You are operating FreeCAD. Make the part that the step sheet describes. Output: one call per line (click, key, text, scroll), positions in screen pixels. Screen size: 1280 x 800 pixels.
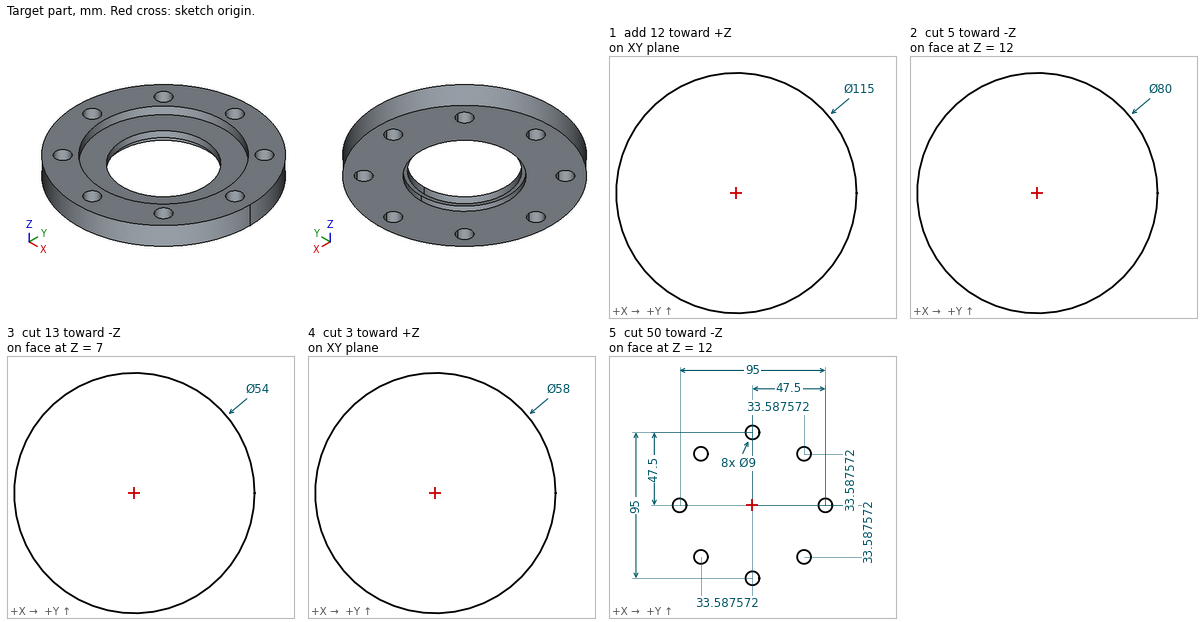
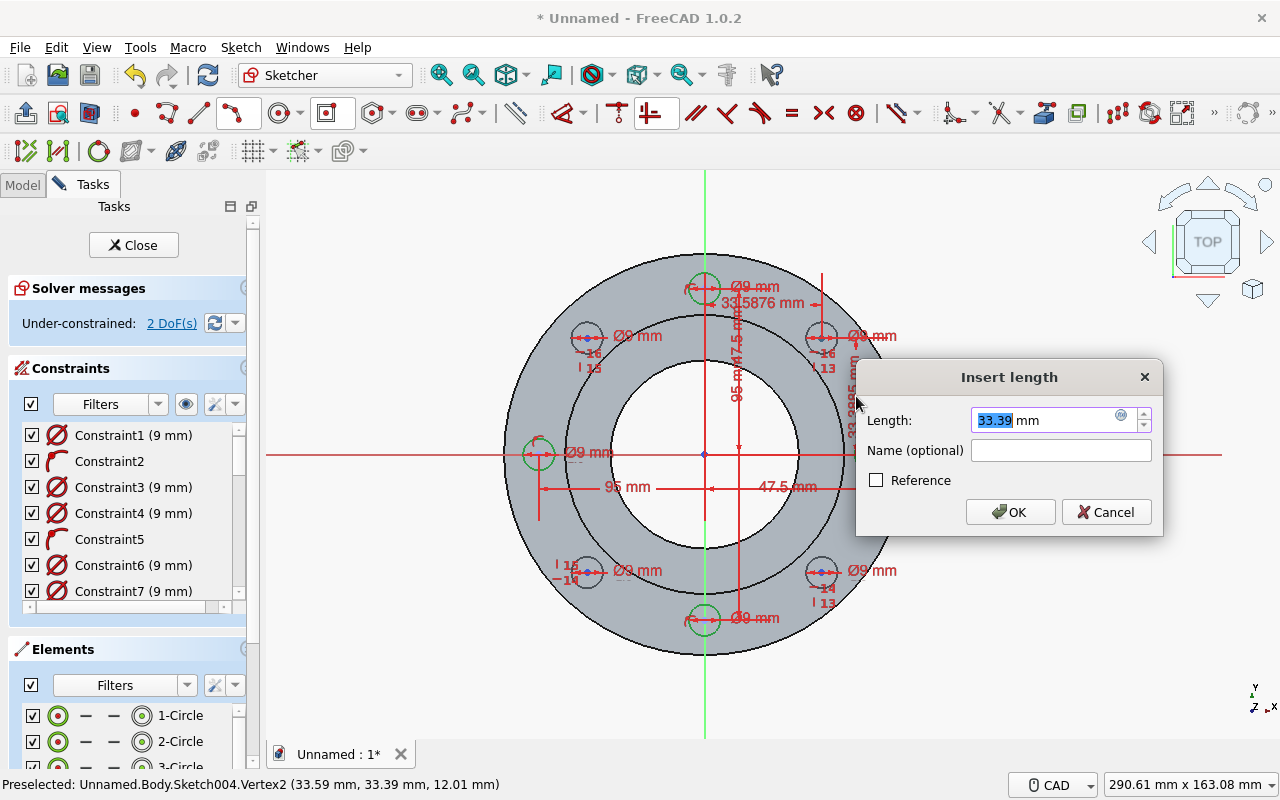
text(33.587572)
key(Return)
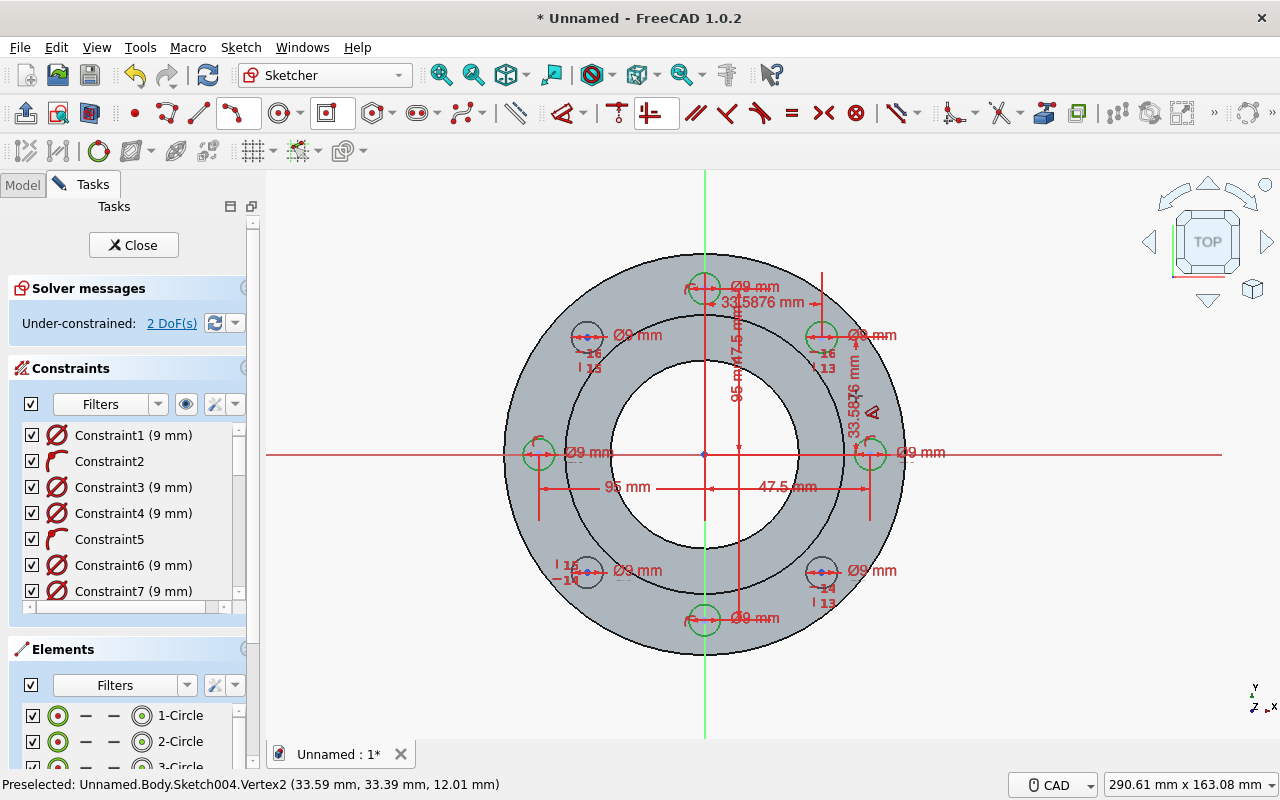
click(822, 573)
click(856, 514)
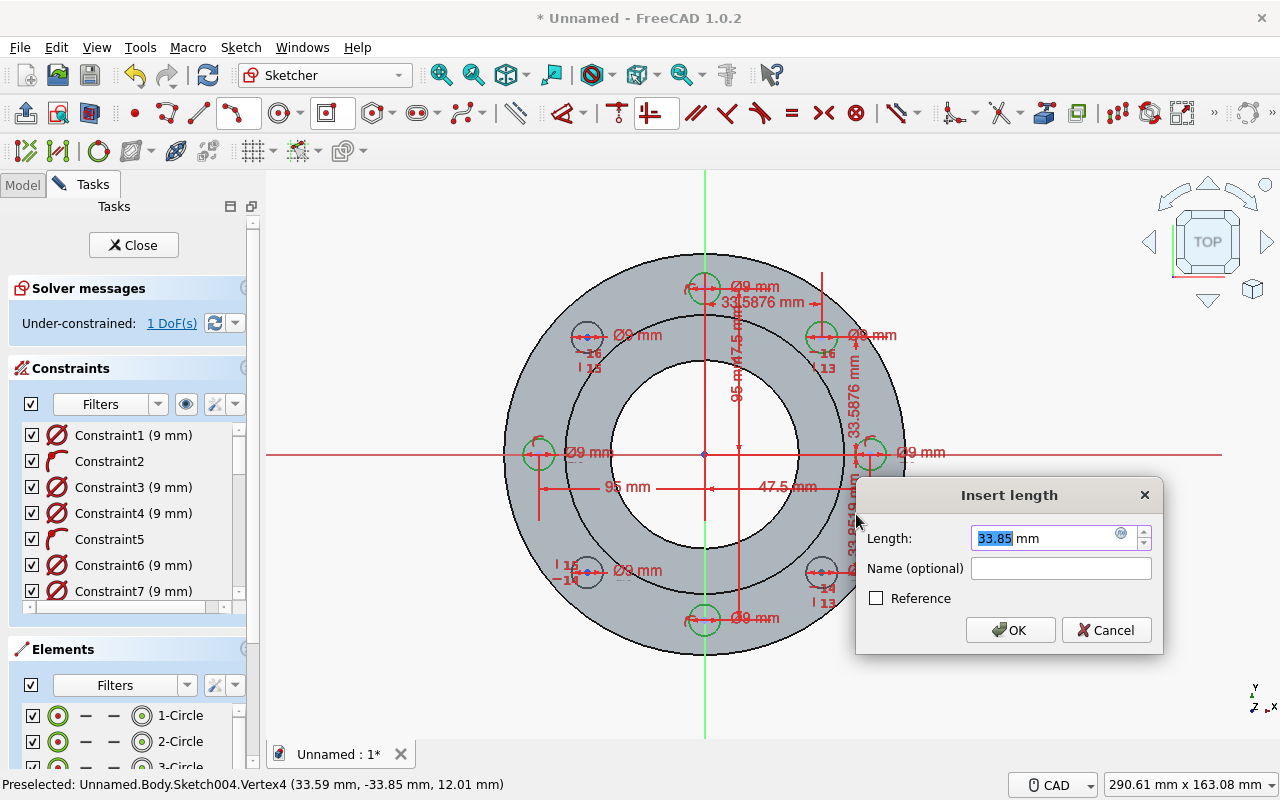
text(33.587572)
key(Return)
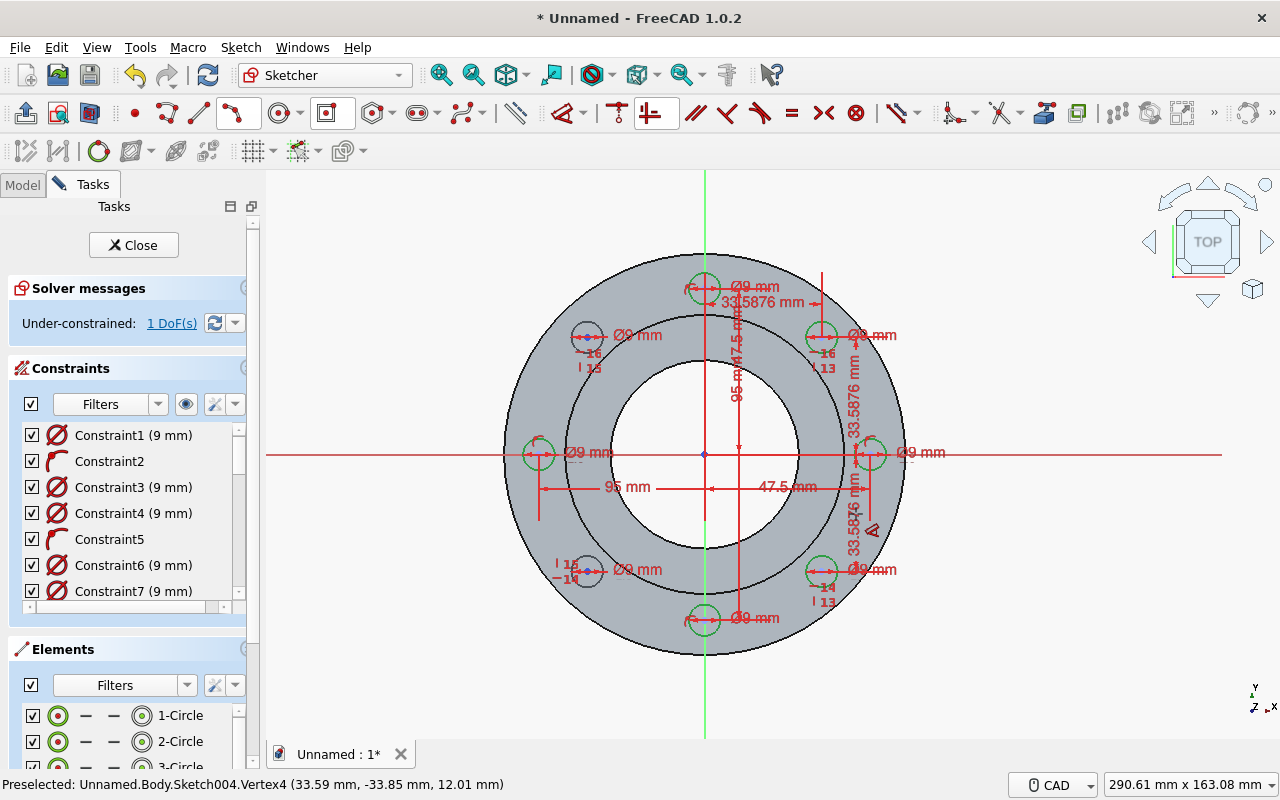
click(587, 572)
click(646, 606)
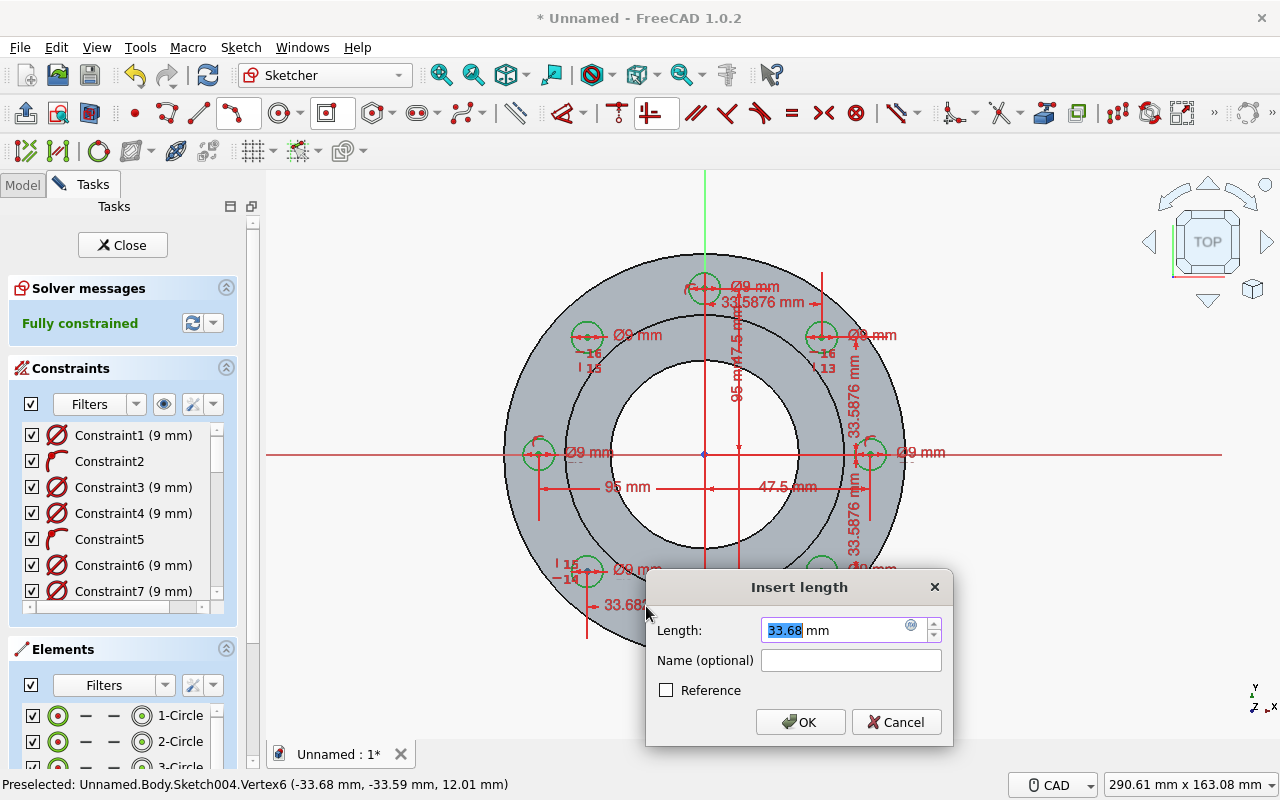
text(33.587572)
key(Return)
key(Escape)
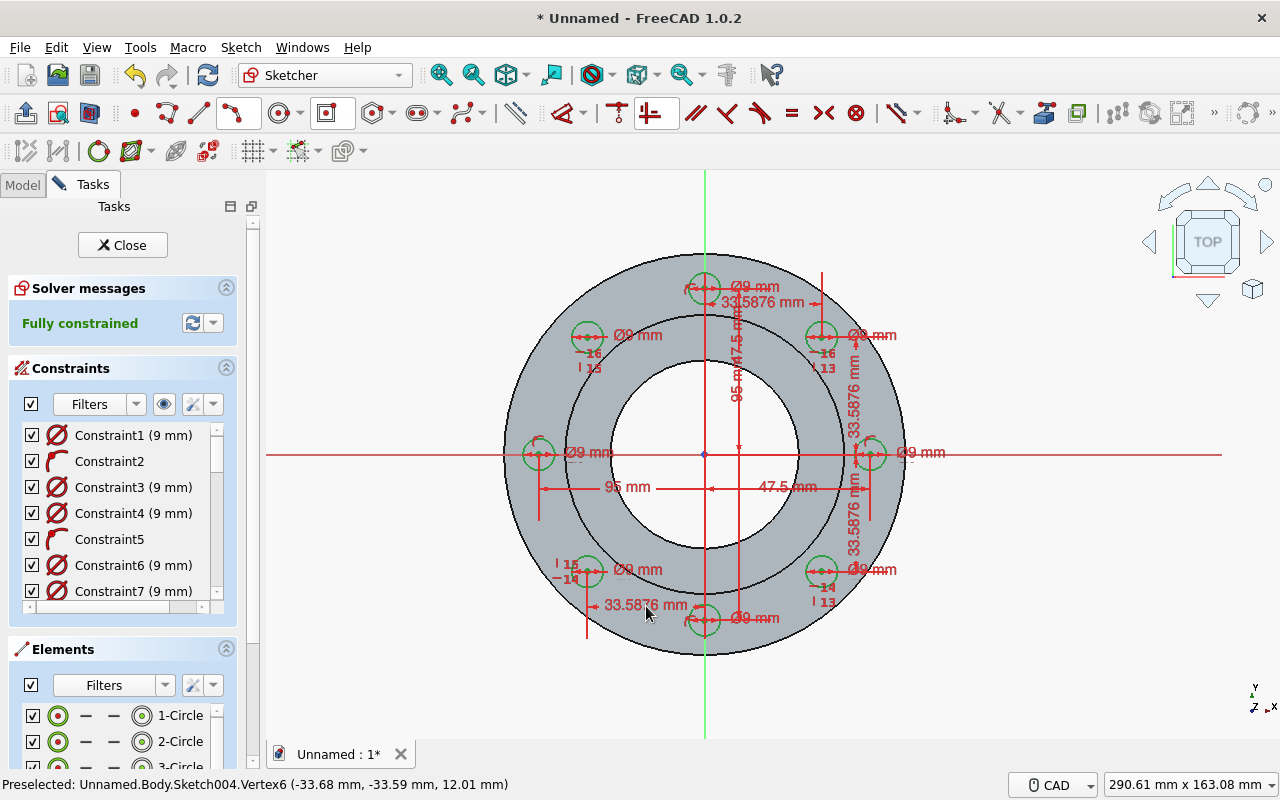
click(123, 245)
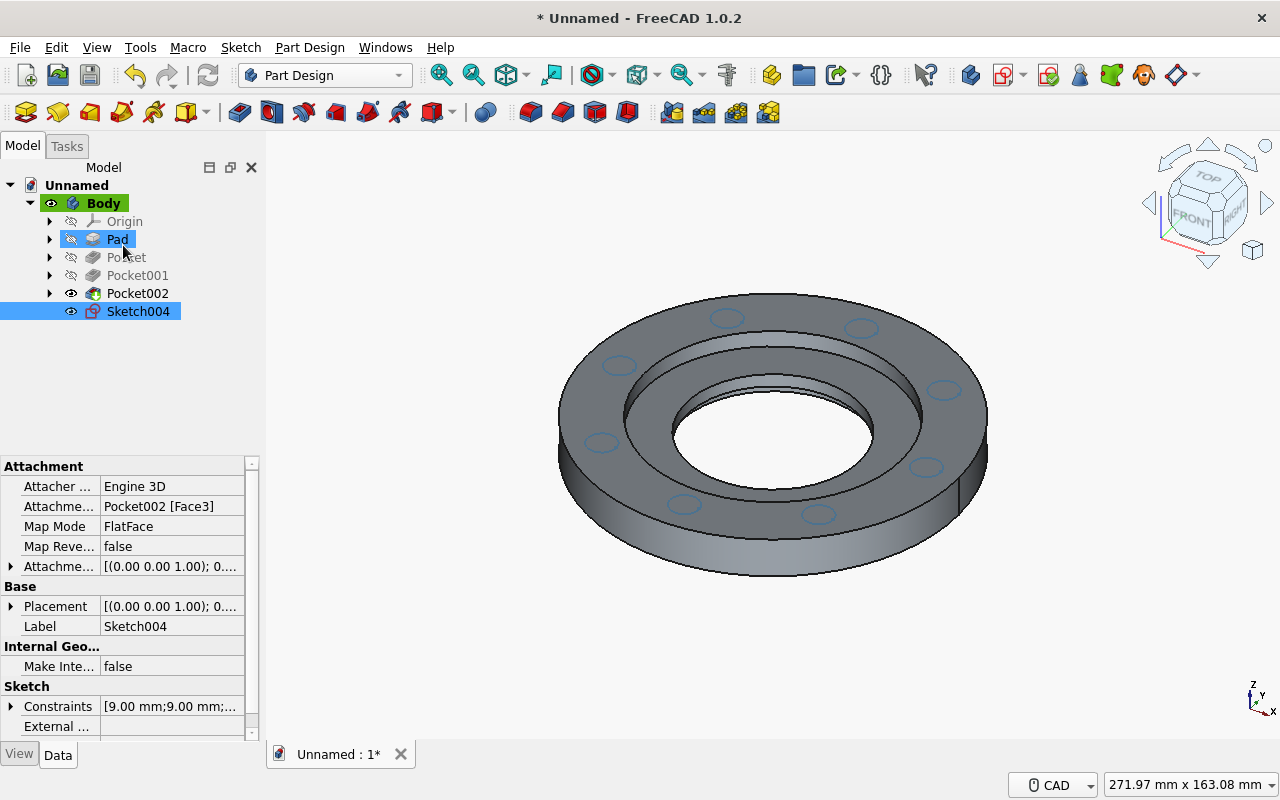
click(240, 112)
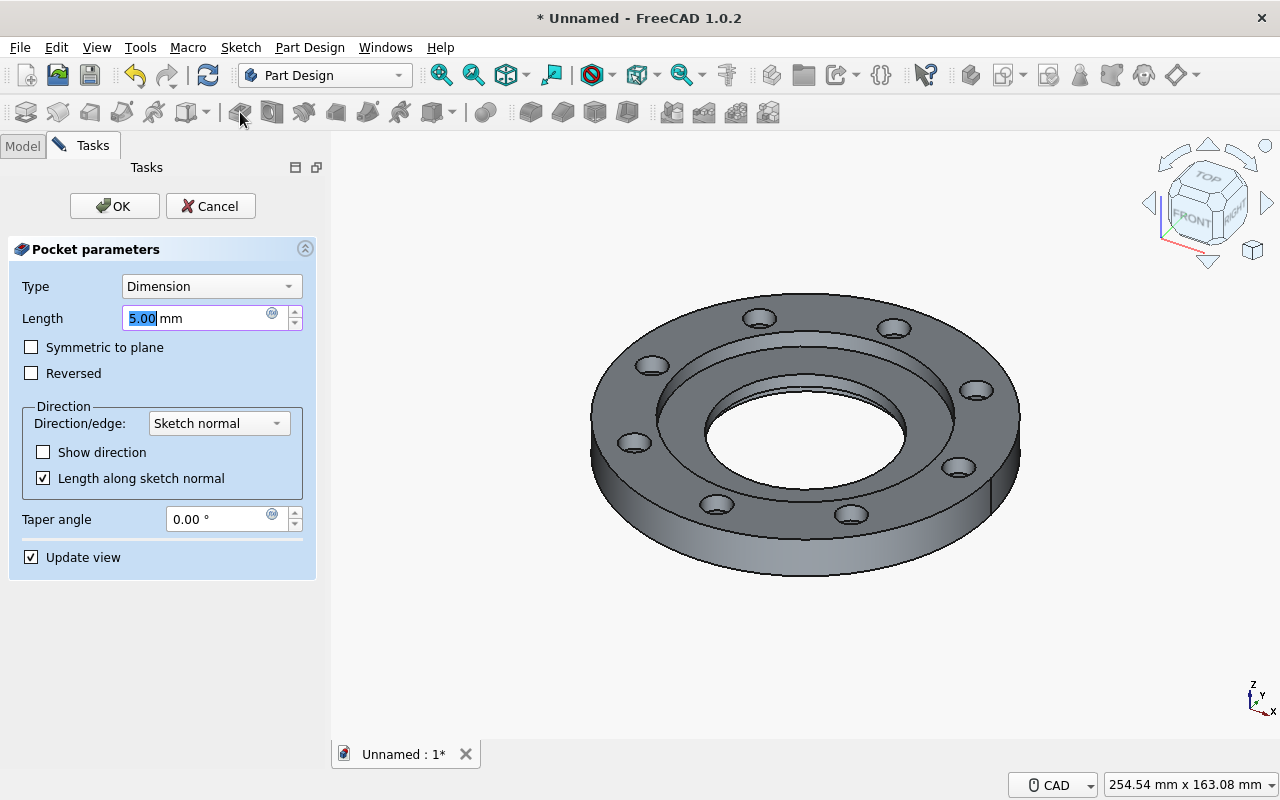
text(50)
key(Tab)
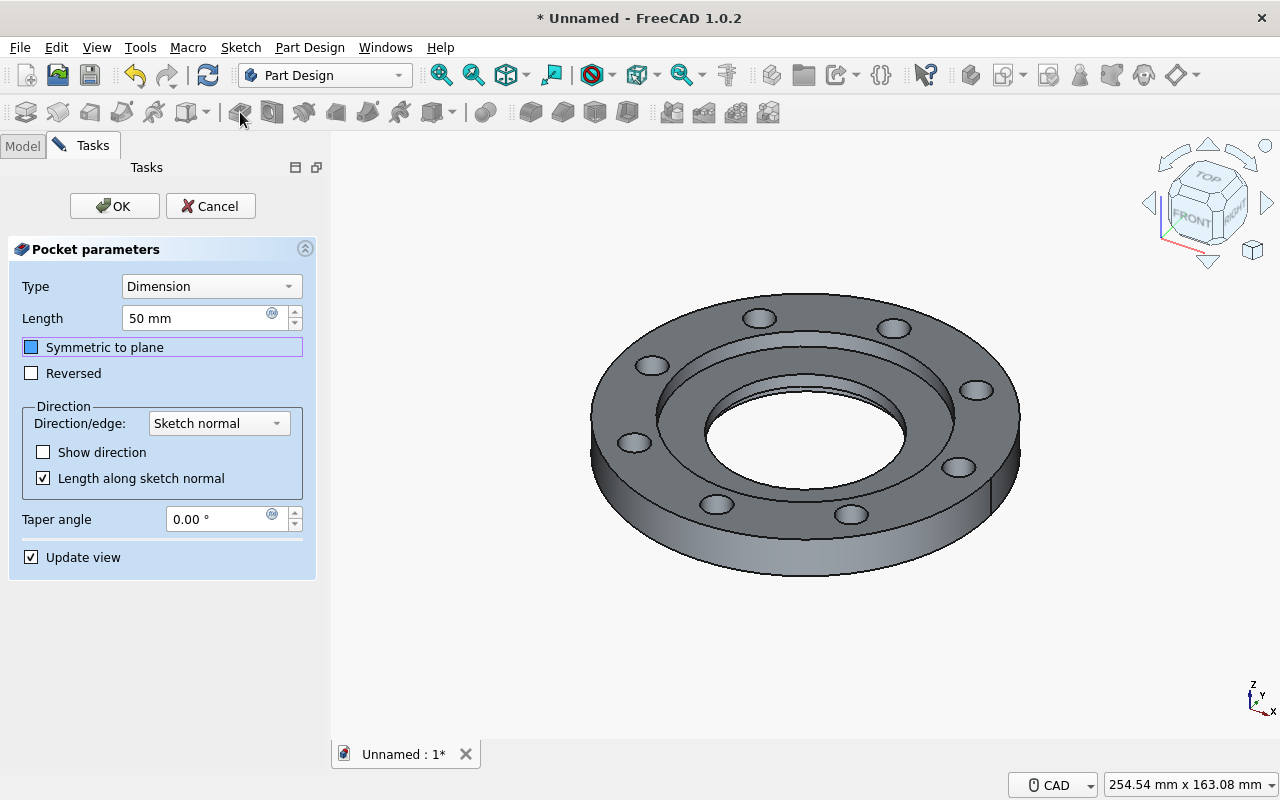
click(115, 206)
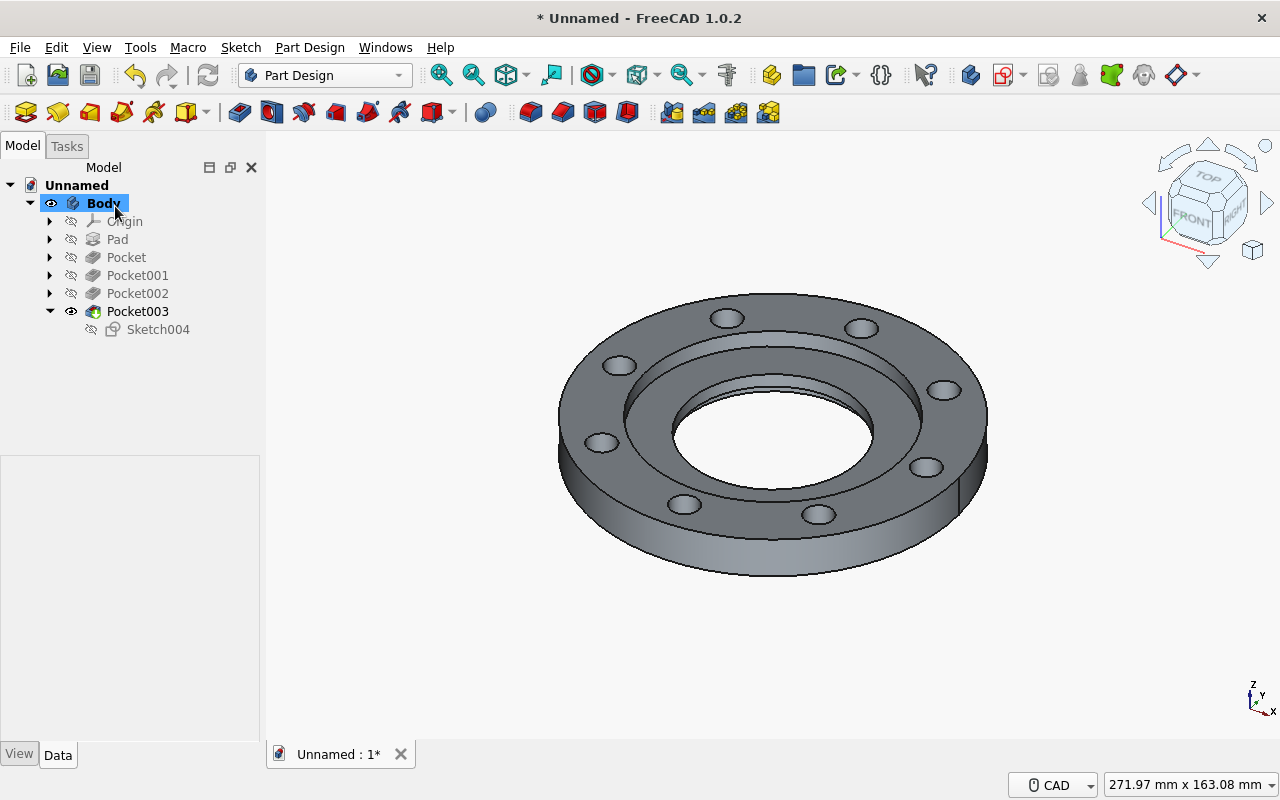
key(0)